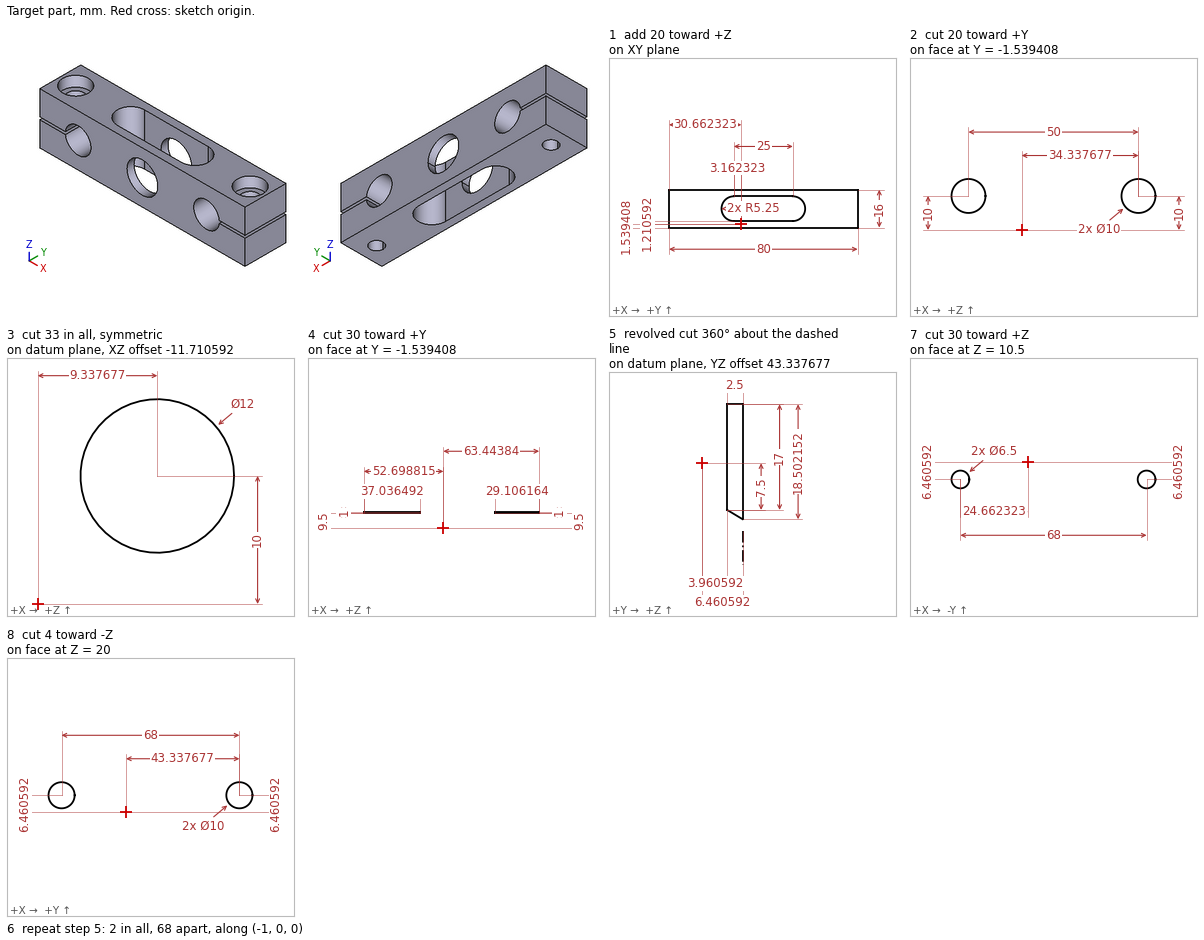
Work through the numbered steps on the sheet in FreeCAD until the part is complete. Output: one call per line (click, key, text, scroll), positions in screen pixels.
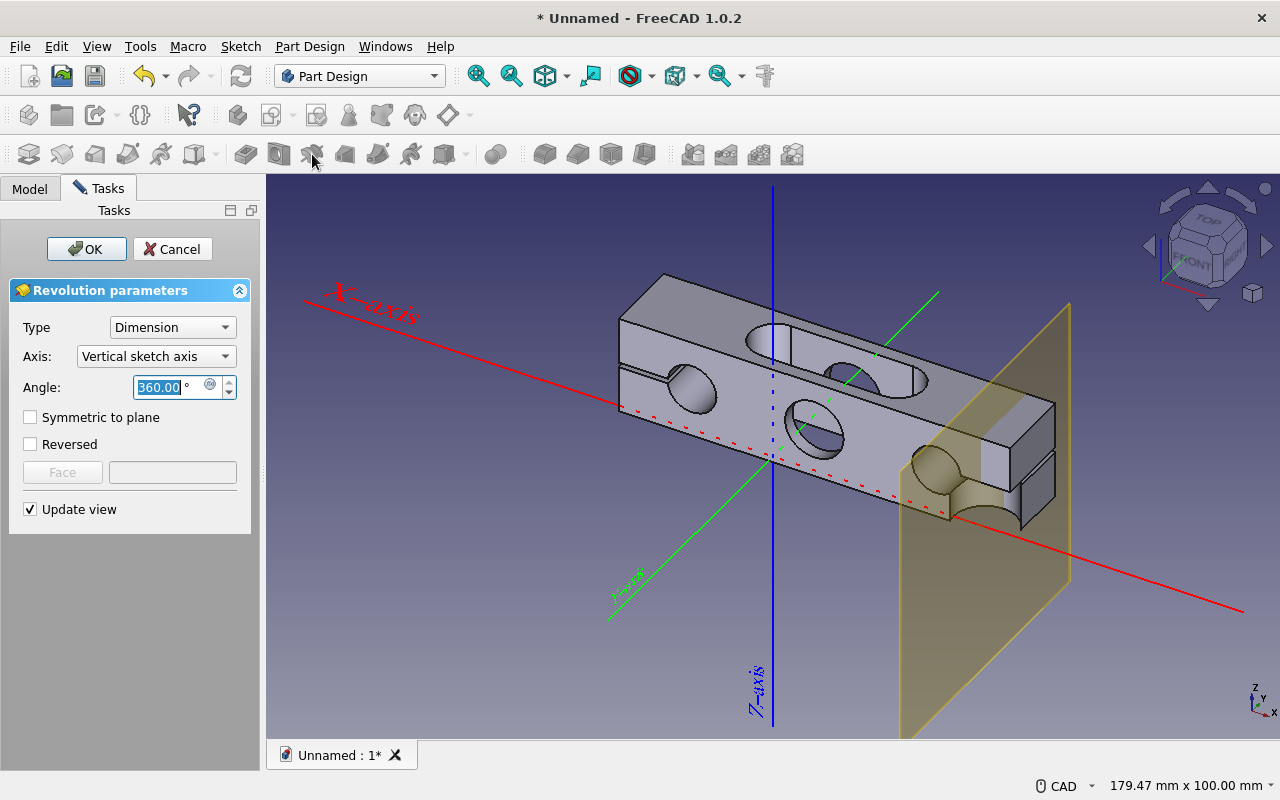
click(157, 356)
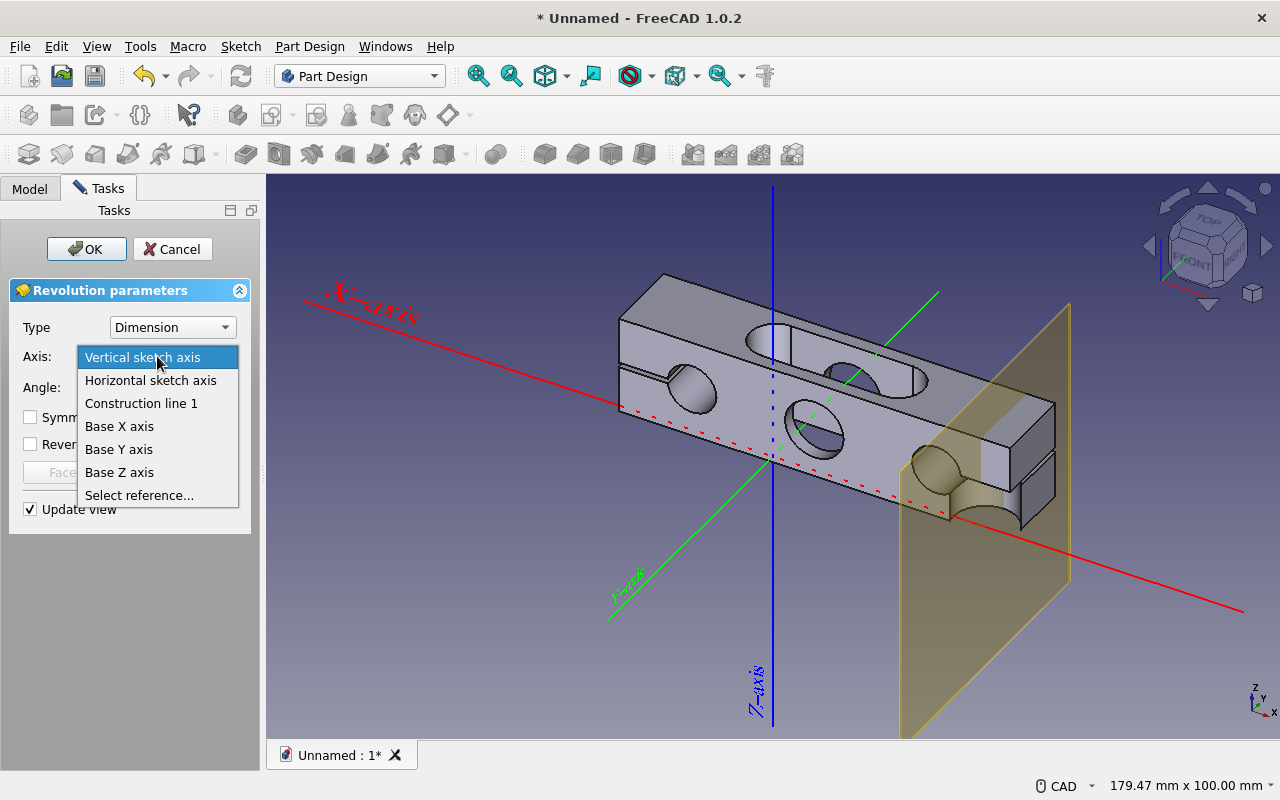
click(156, 404)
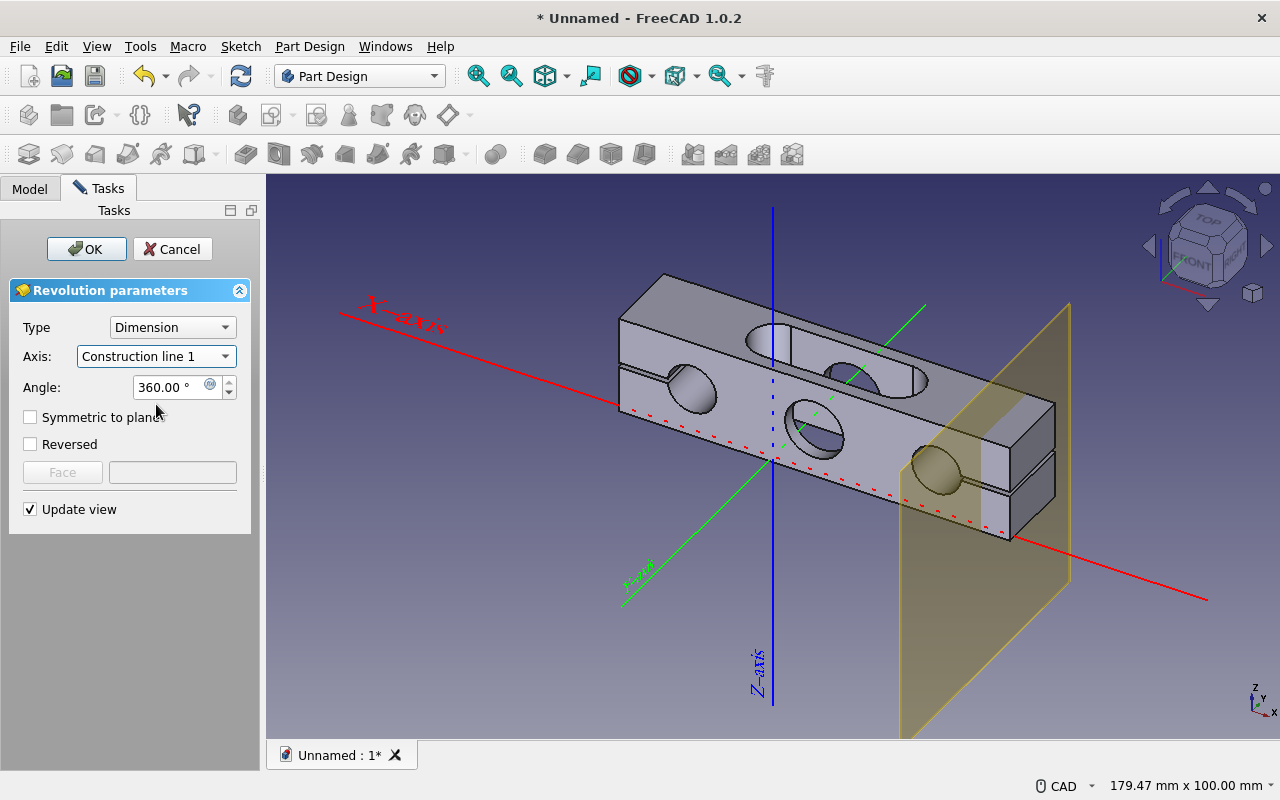
click(87, 249)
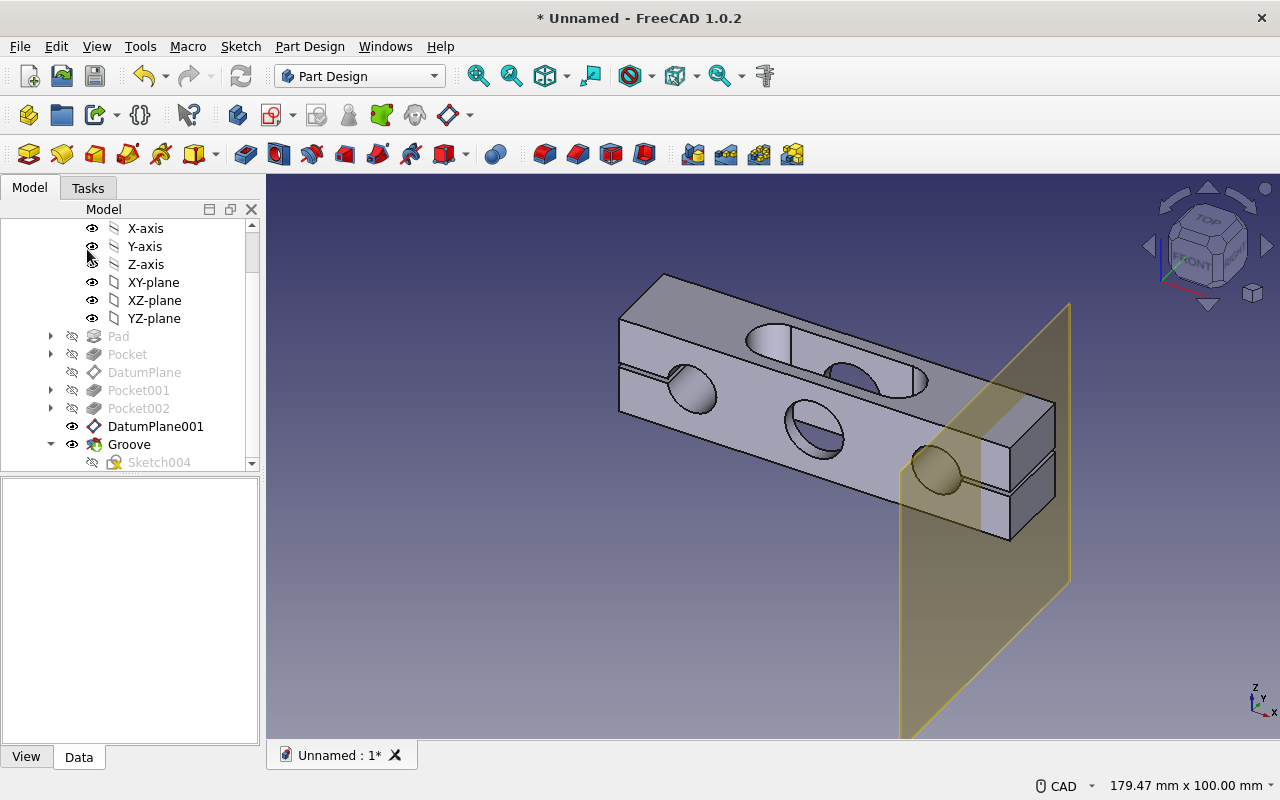
click(117, 426)
key(space)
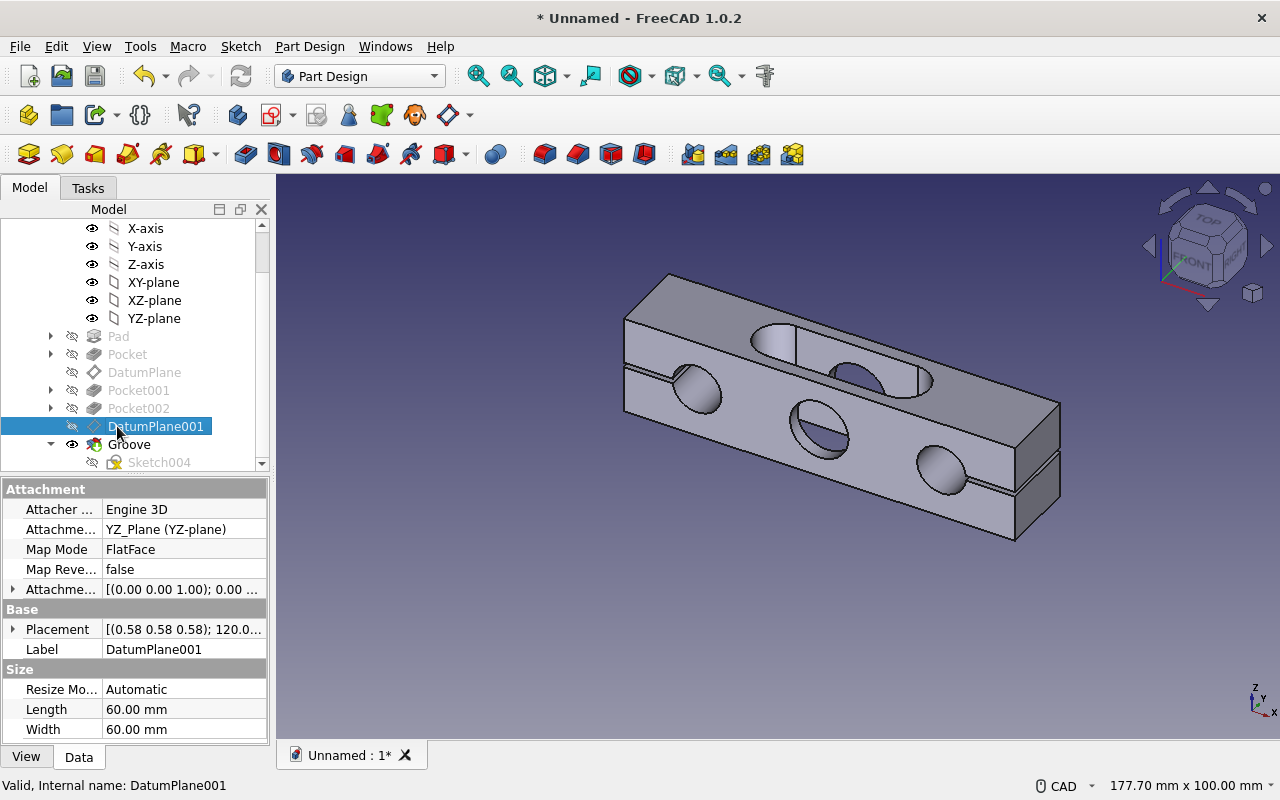
click(117, 444)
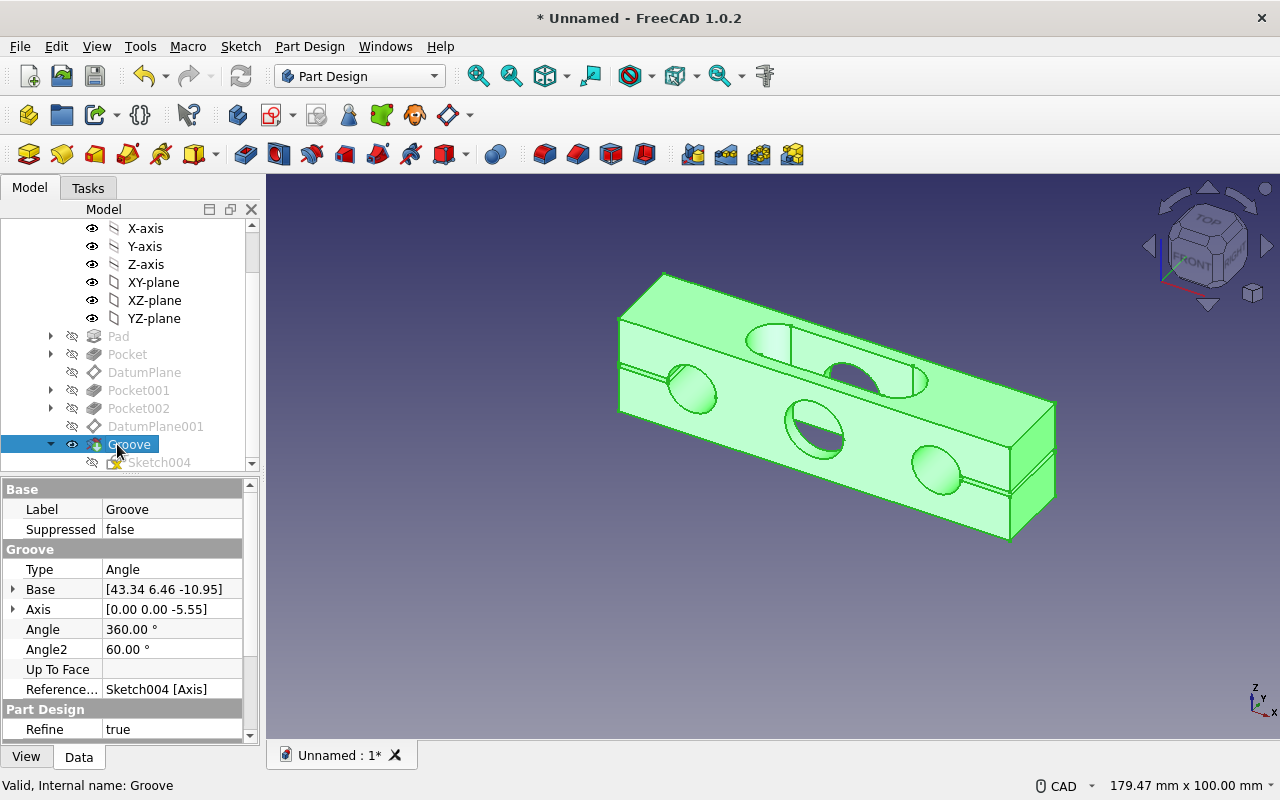
click(726, 154)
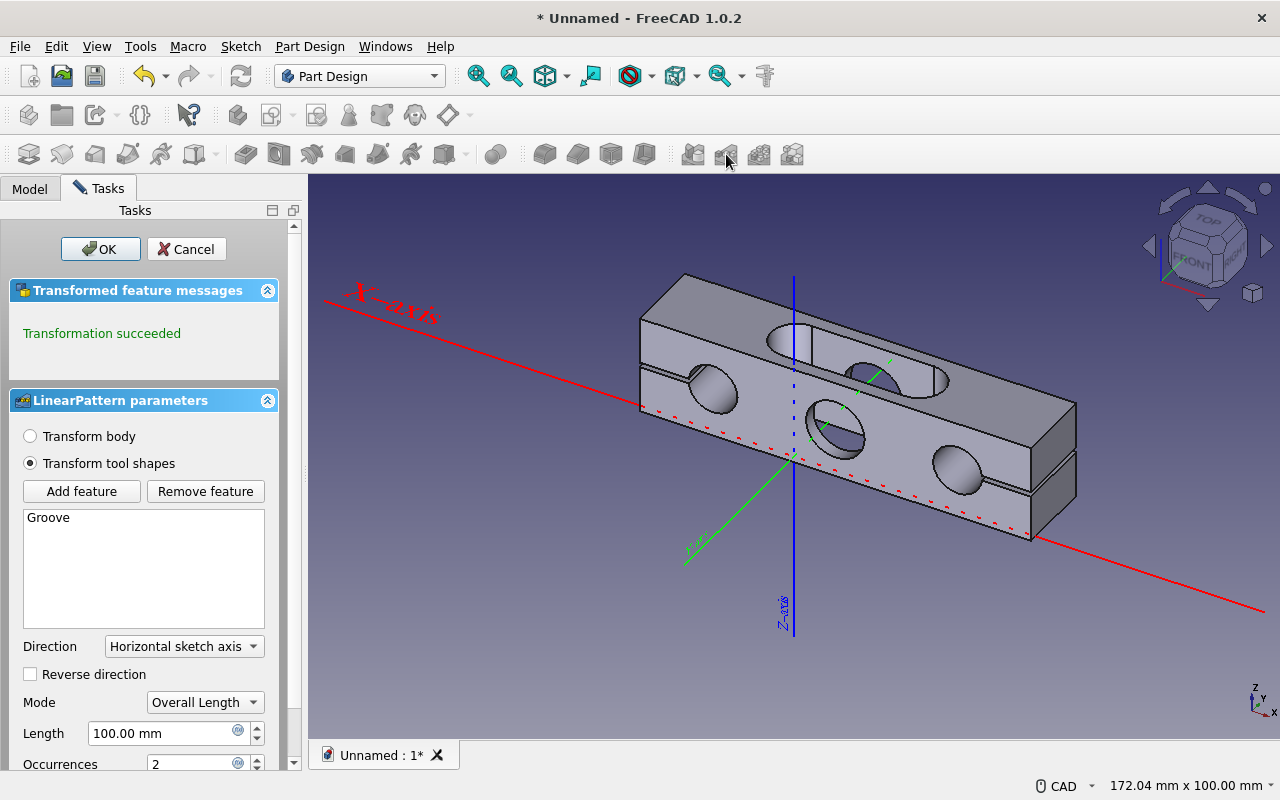
click(185, 646)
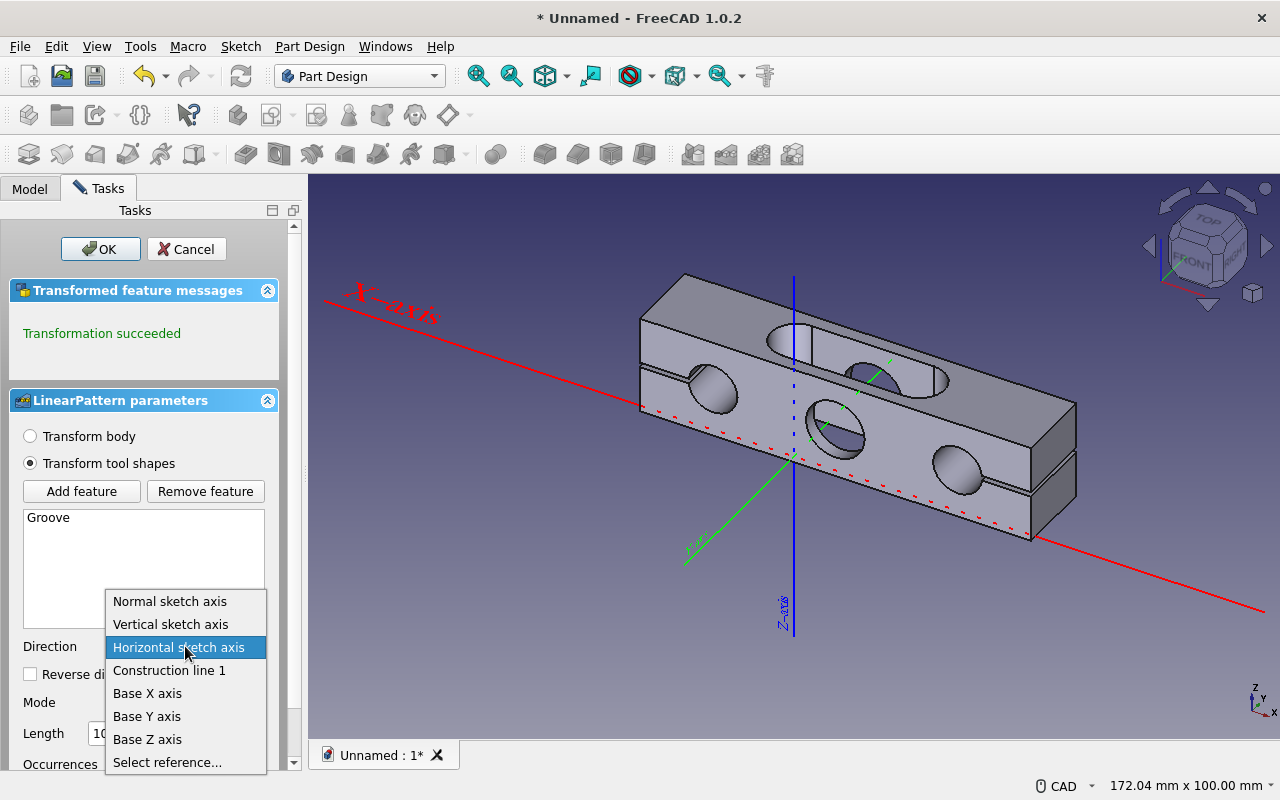
click(184, 694)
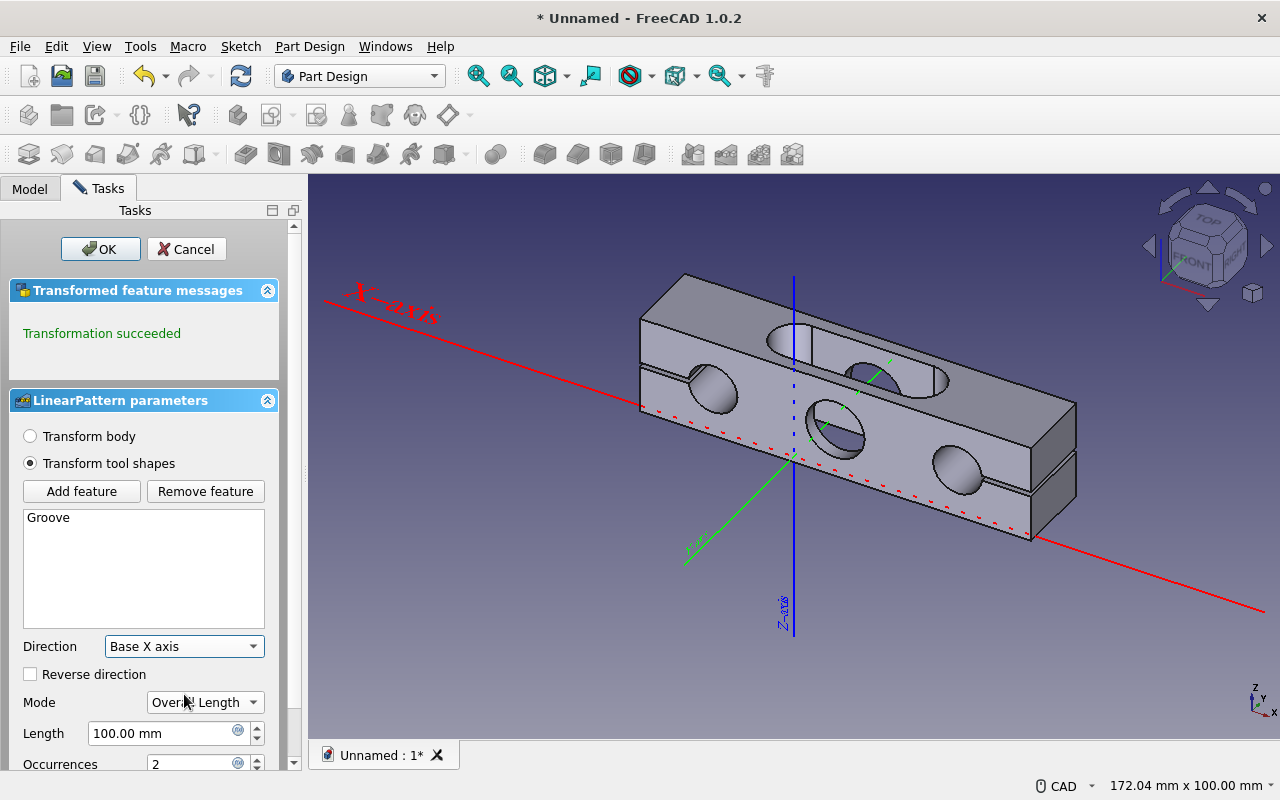
click(206, 702)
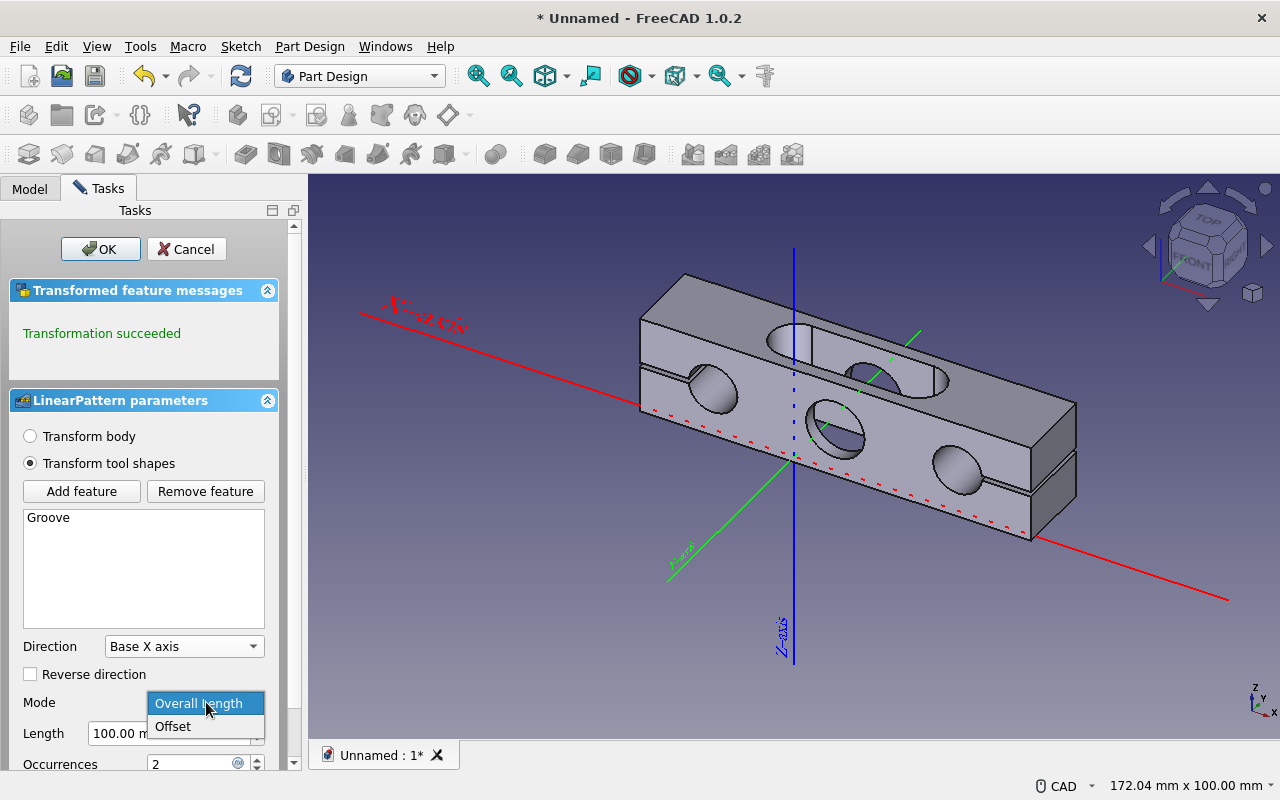
click(204, 726)